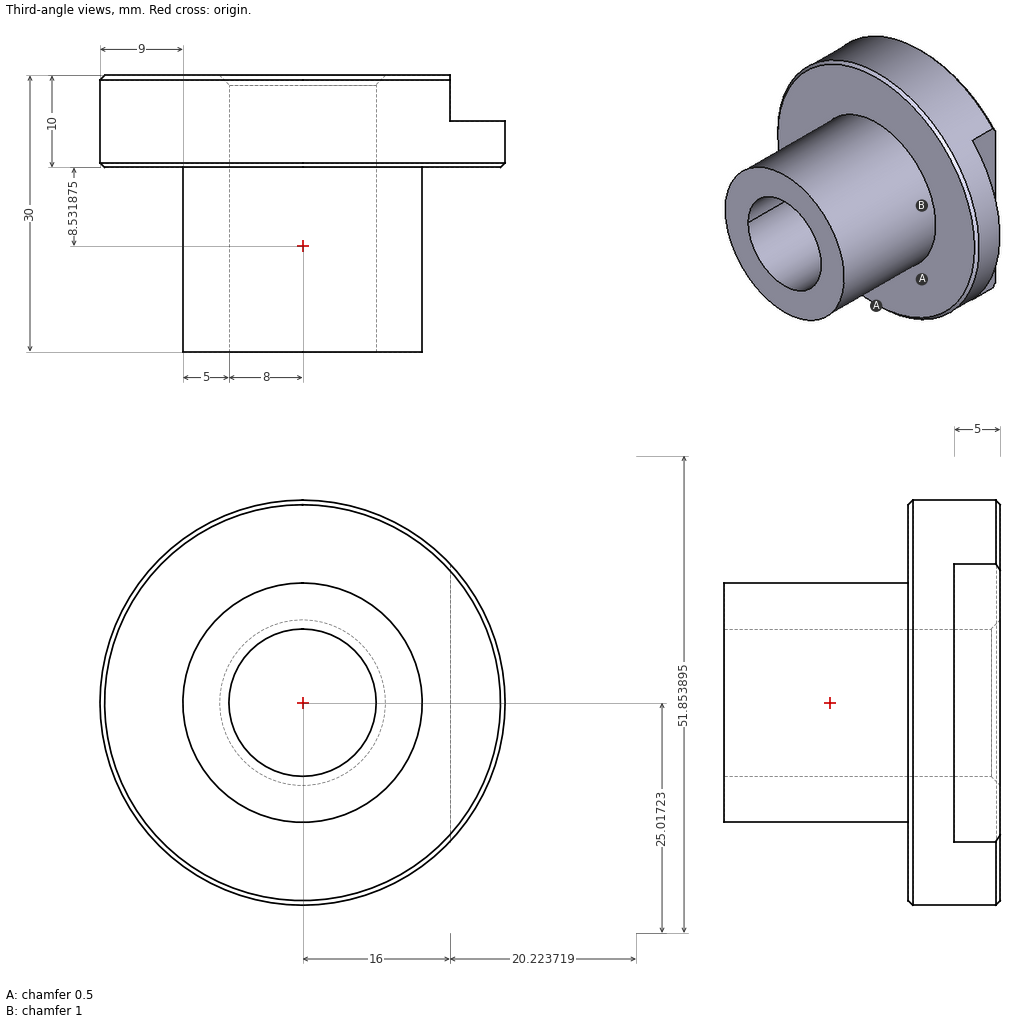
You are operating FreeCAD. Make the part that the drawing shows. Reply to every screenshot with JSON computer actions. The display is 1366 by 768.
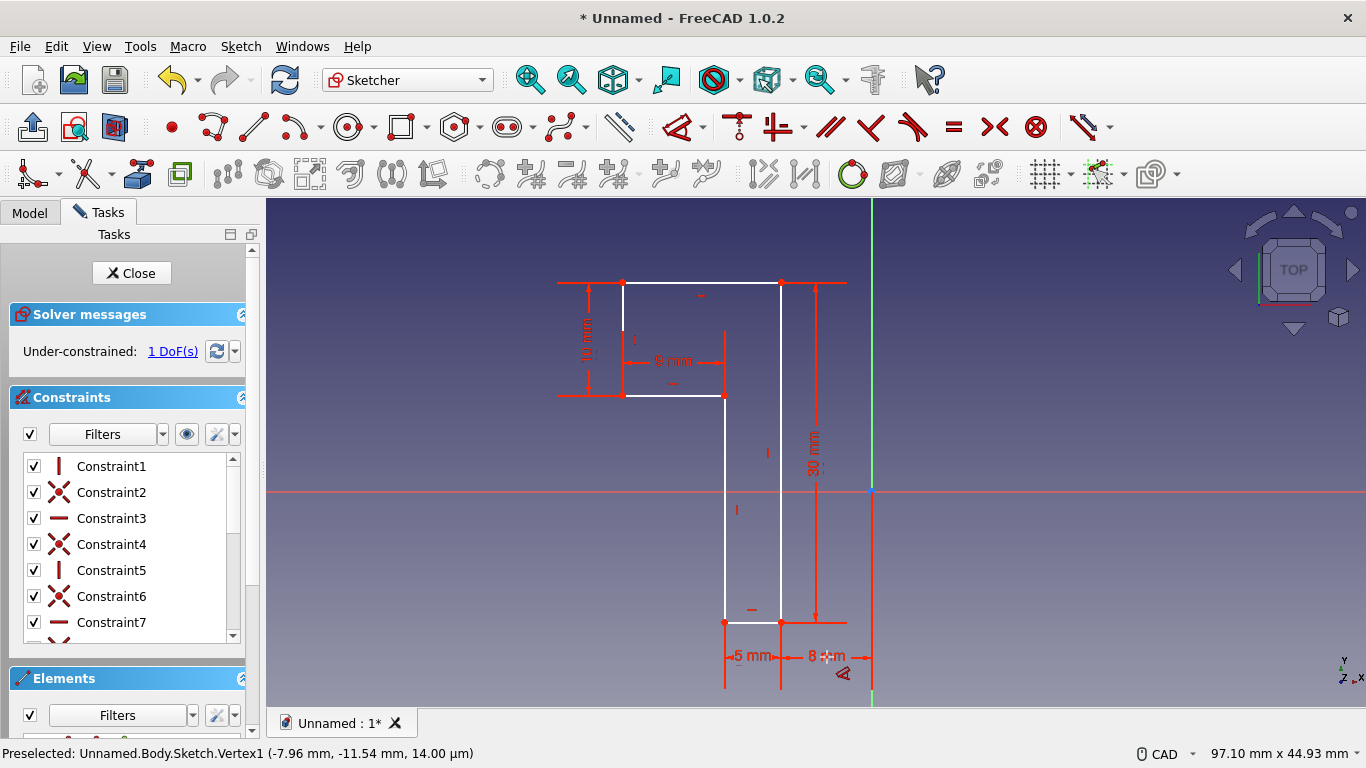
{"action": "left_click", "coordinate": [623, 396]}
{"action": "left_click", "coordinate": [906, 444]}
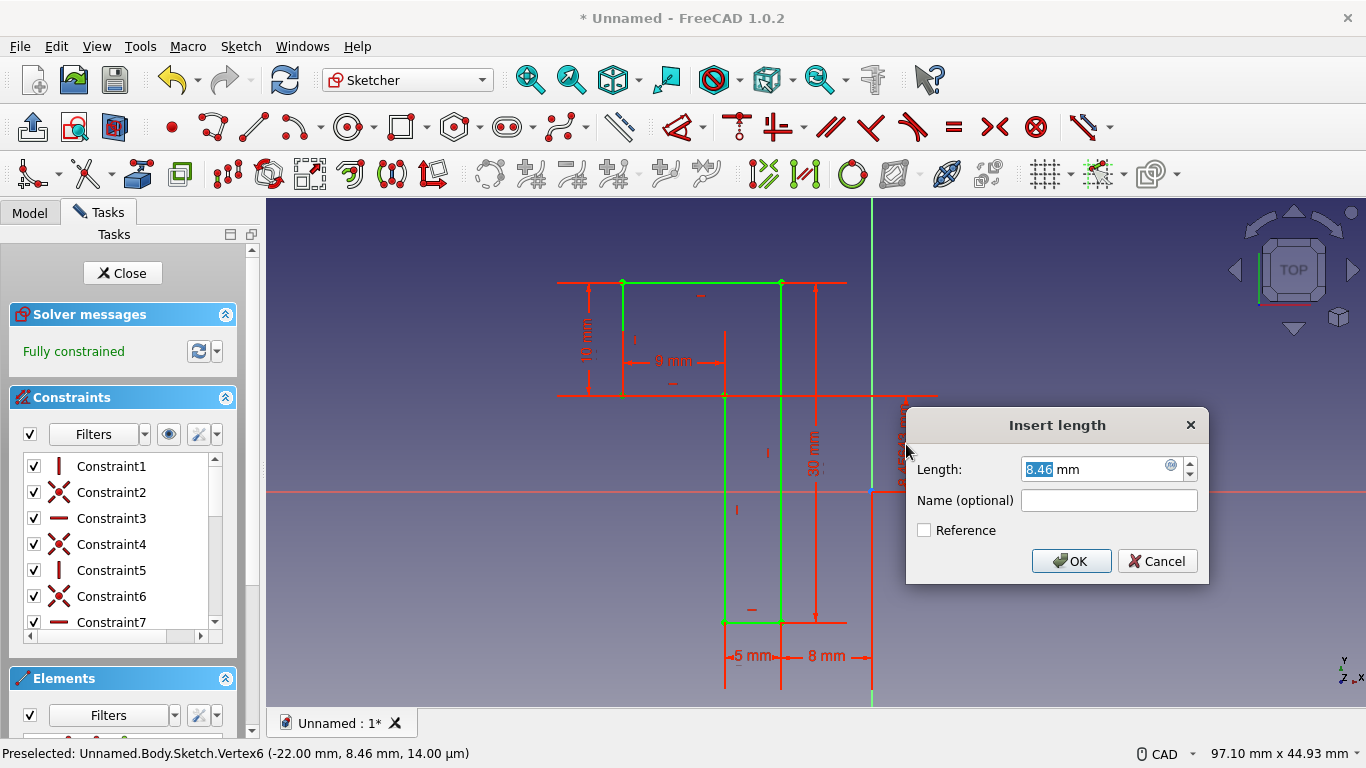
{"action": "type", "text": "8.531875"}
{"action": "key", "text": "Return"}
{"action": "key", "text": "Escape"}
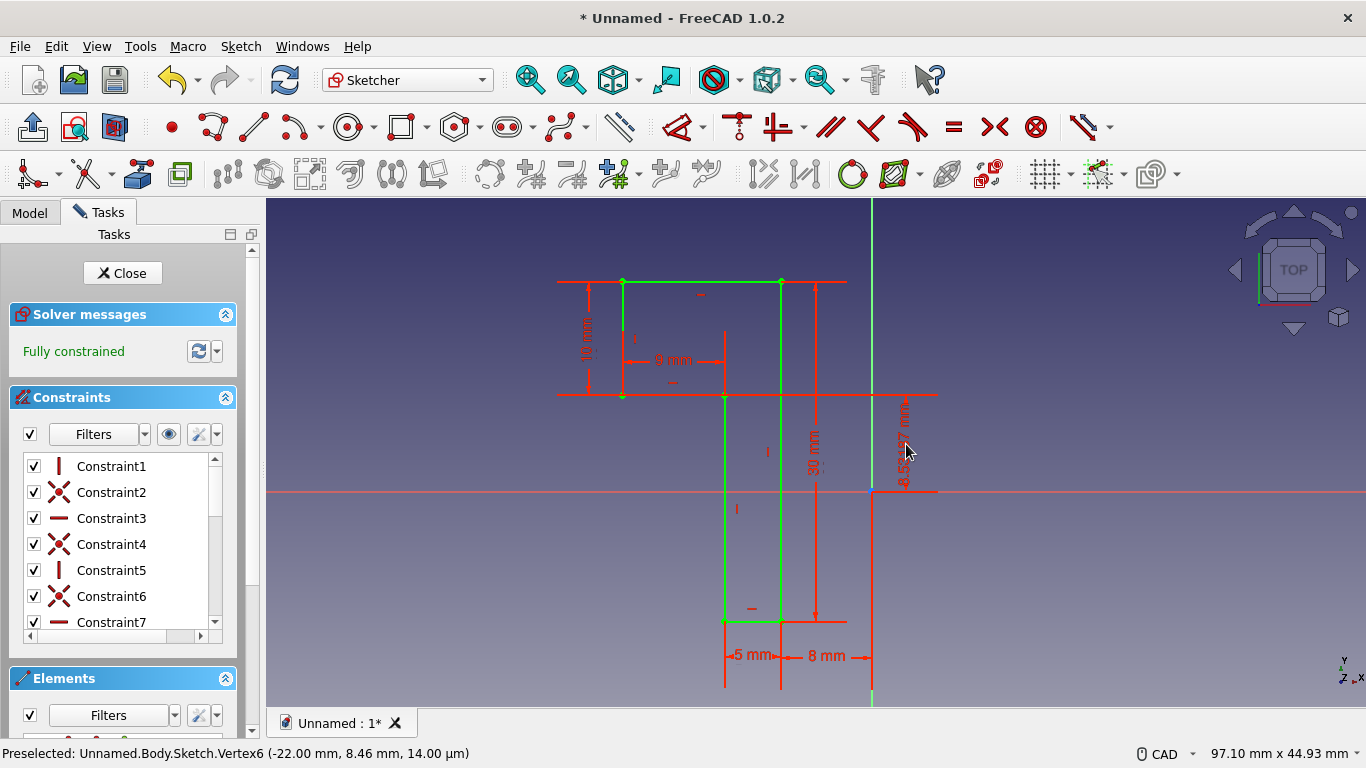
{"action": "left_click", "coordinate": [123, 273]}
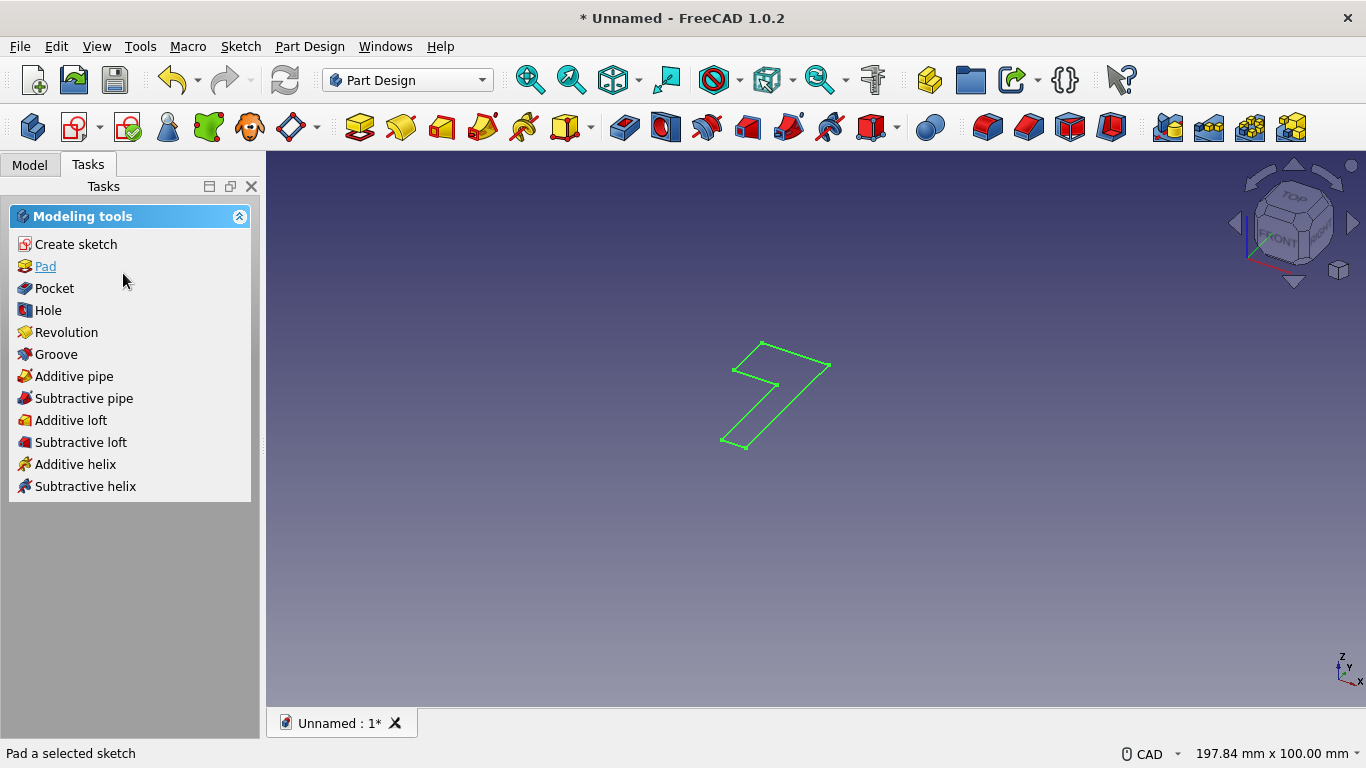
{"action": "left_click", "coordinate": [401, 128]}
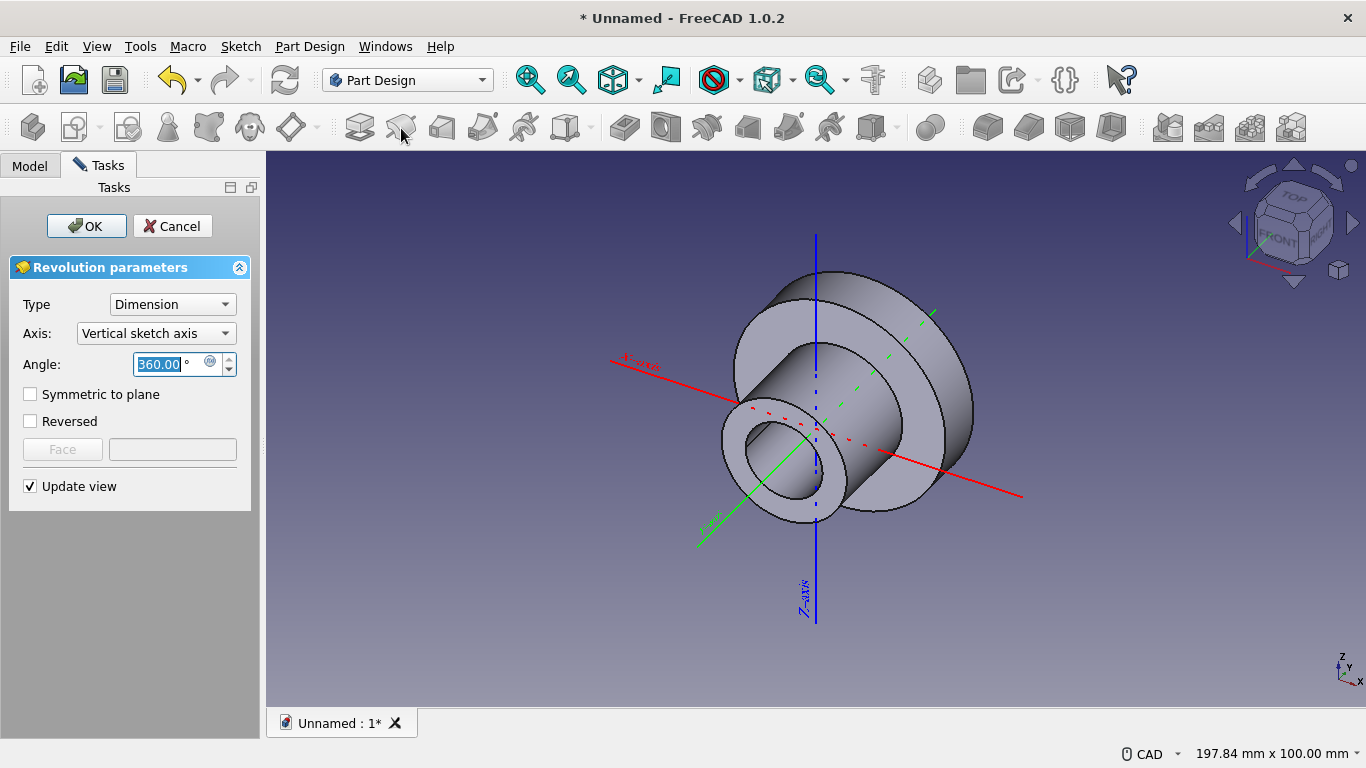
{"action": "left_click", "coordinate": [87, 226]}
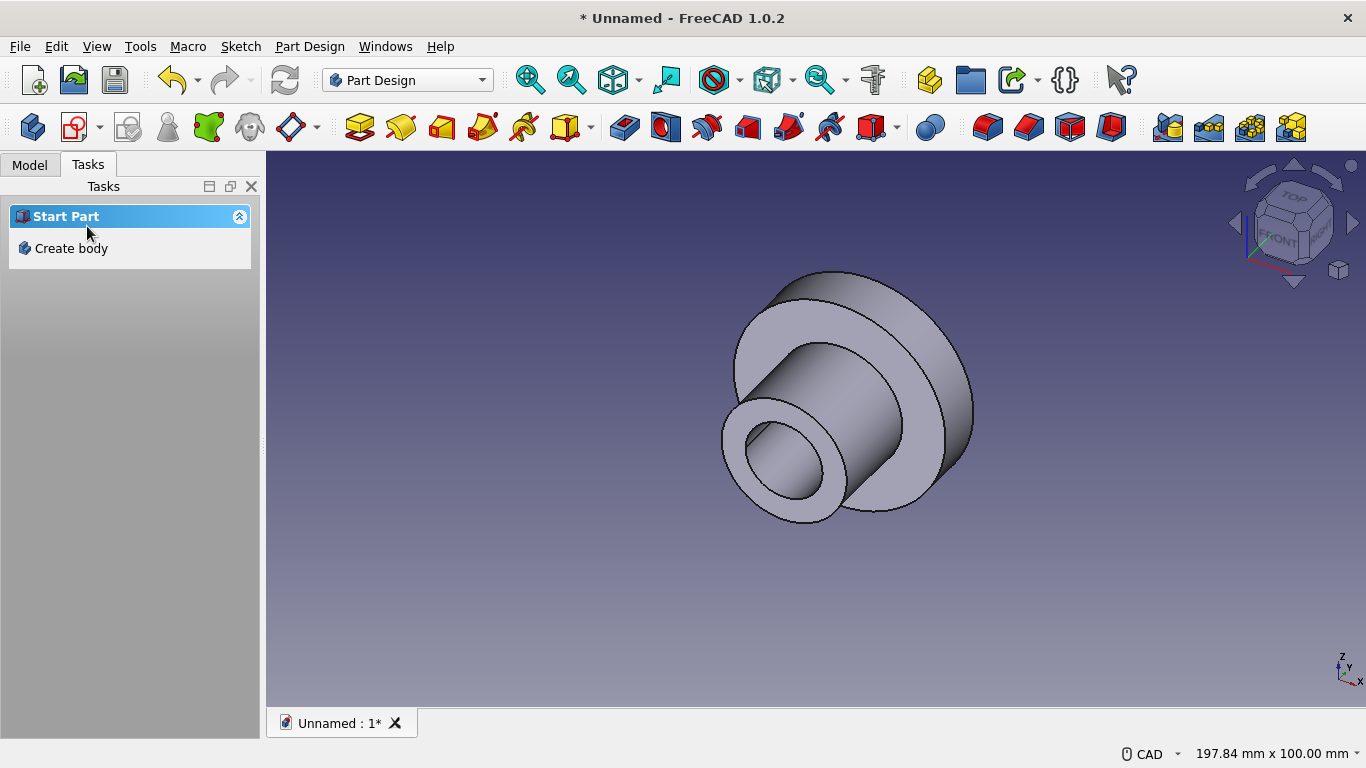
{"action": "left_click", "coordinate": [946, 440]}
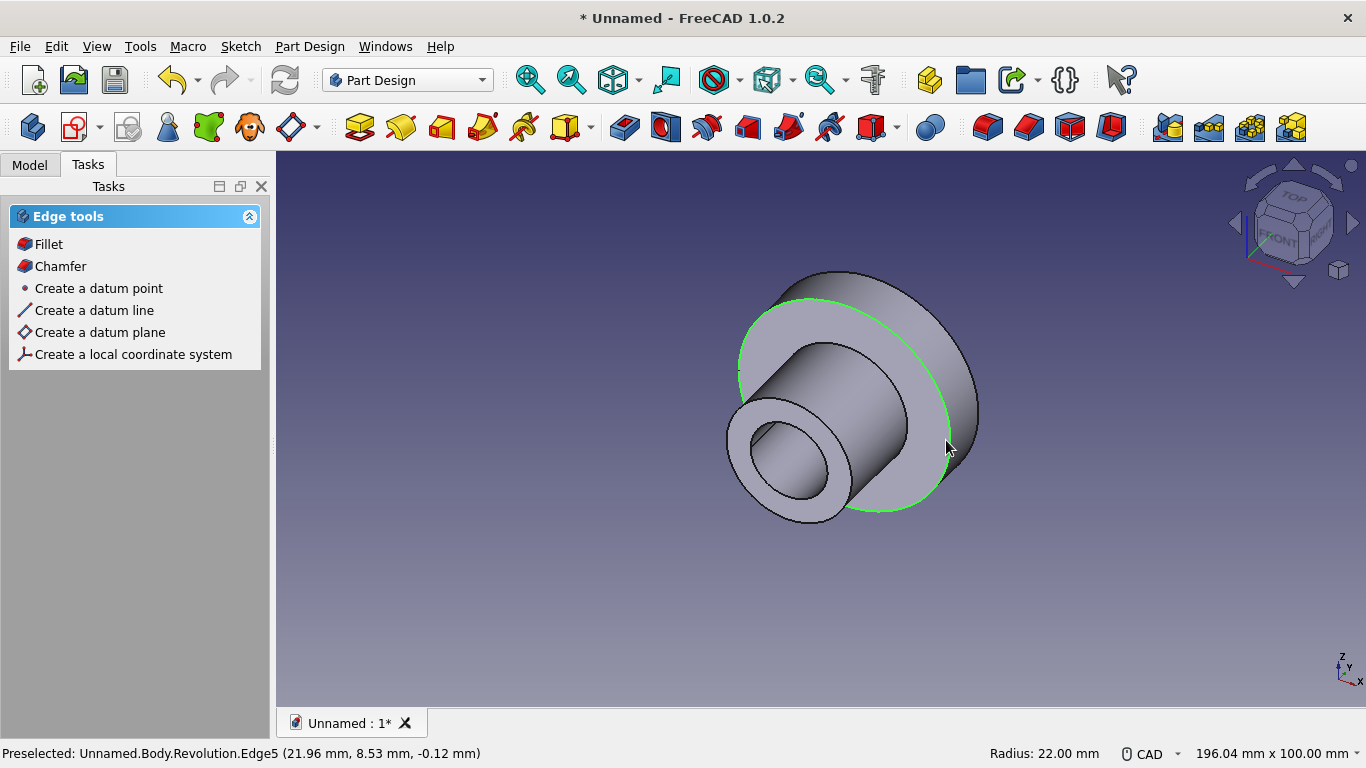
{"action": "key", "text": "0"}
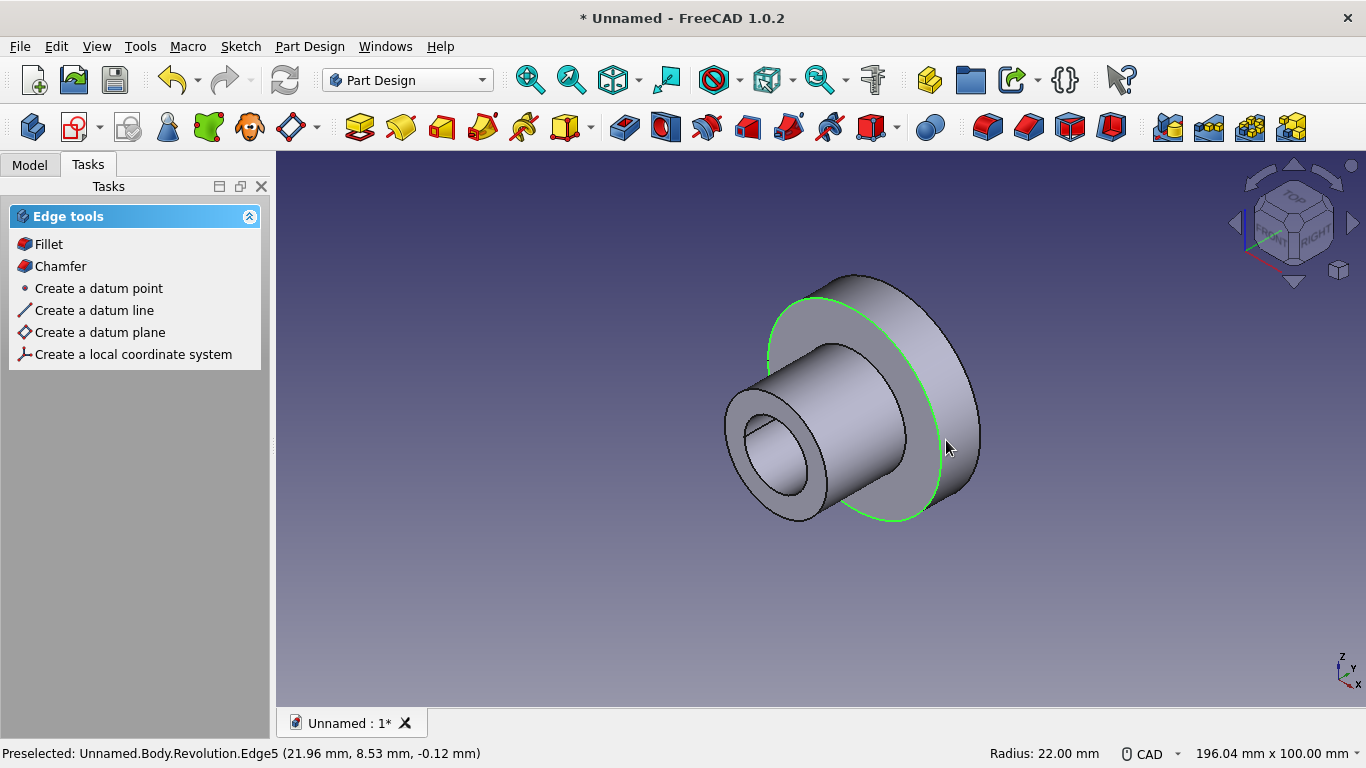
{"action": "key", "text": "2"}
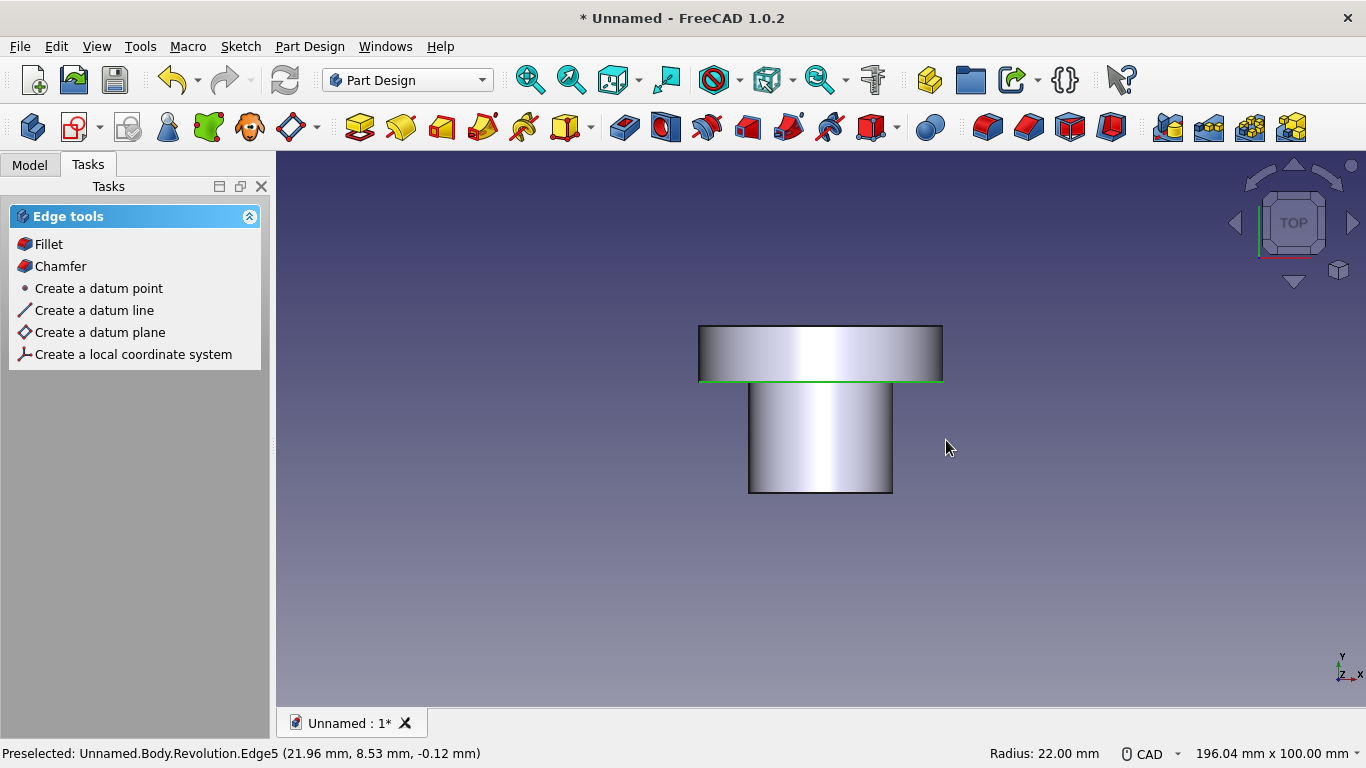
{"action": "left_click", "coordinate": [531, 80]}